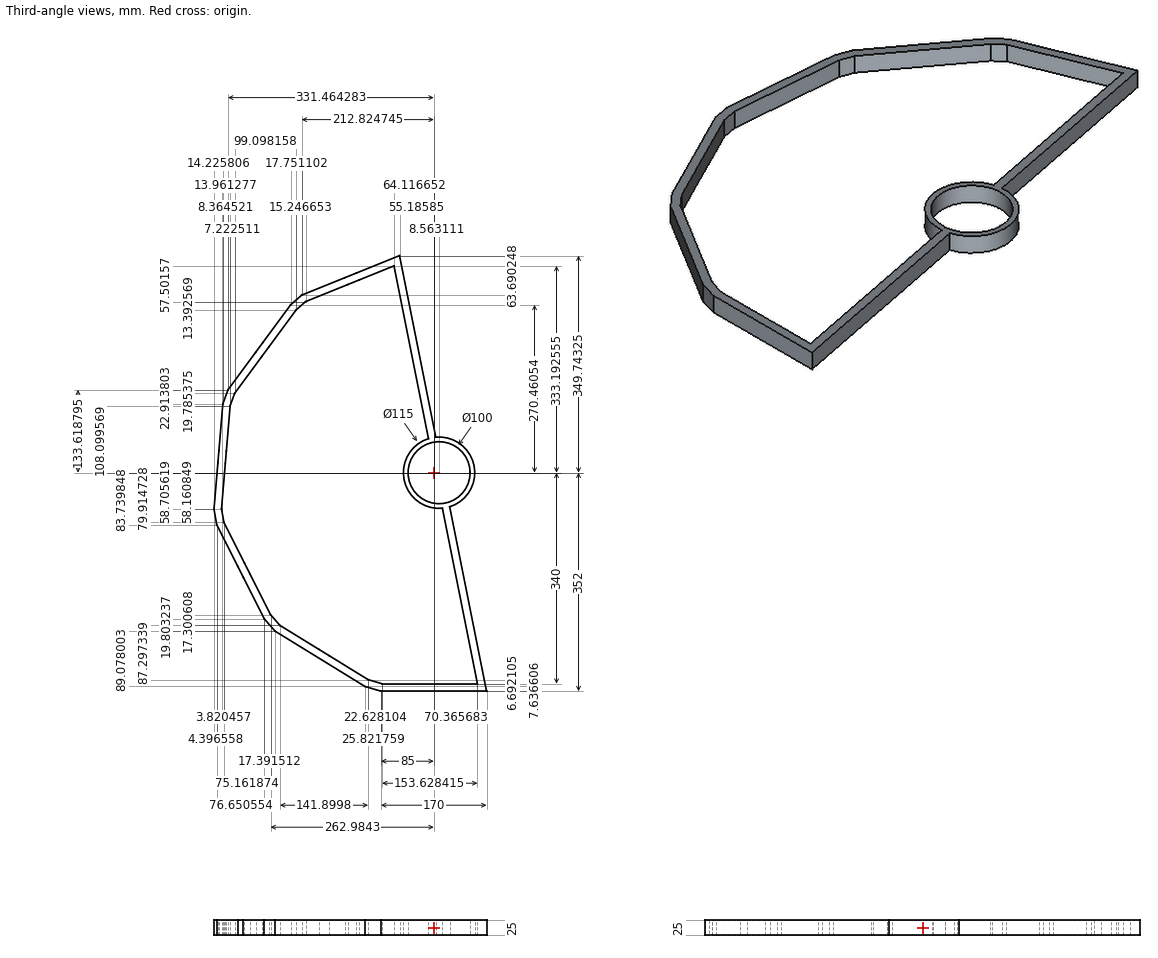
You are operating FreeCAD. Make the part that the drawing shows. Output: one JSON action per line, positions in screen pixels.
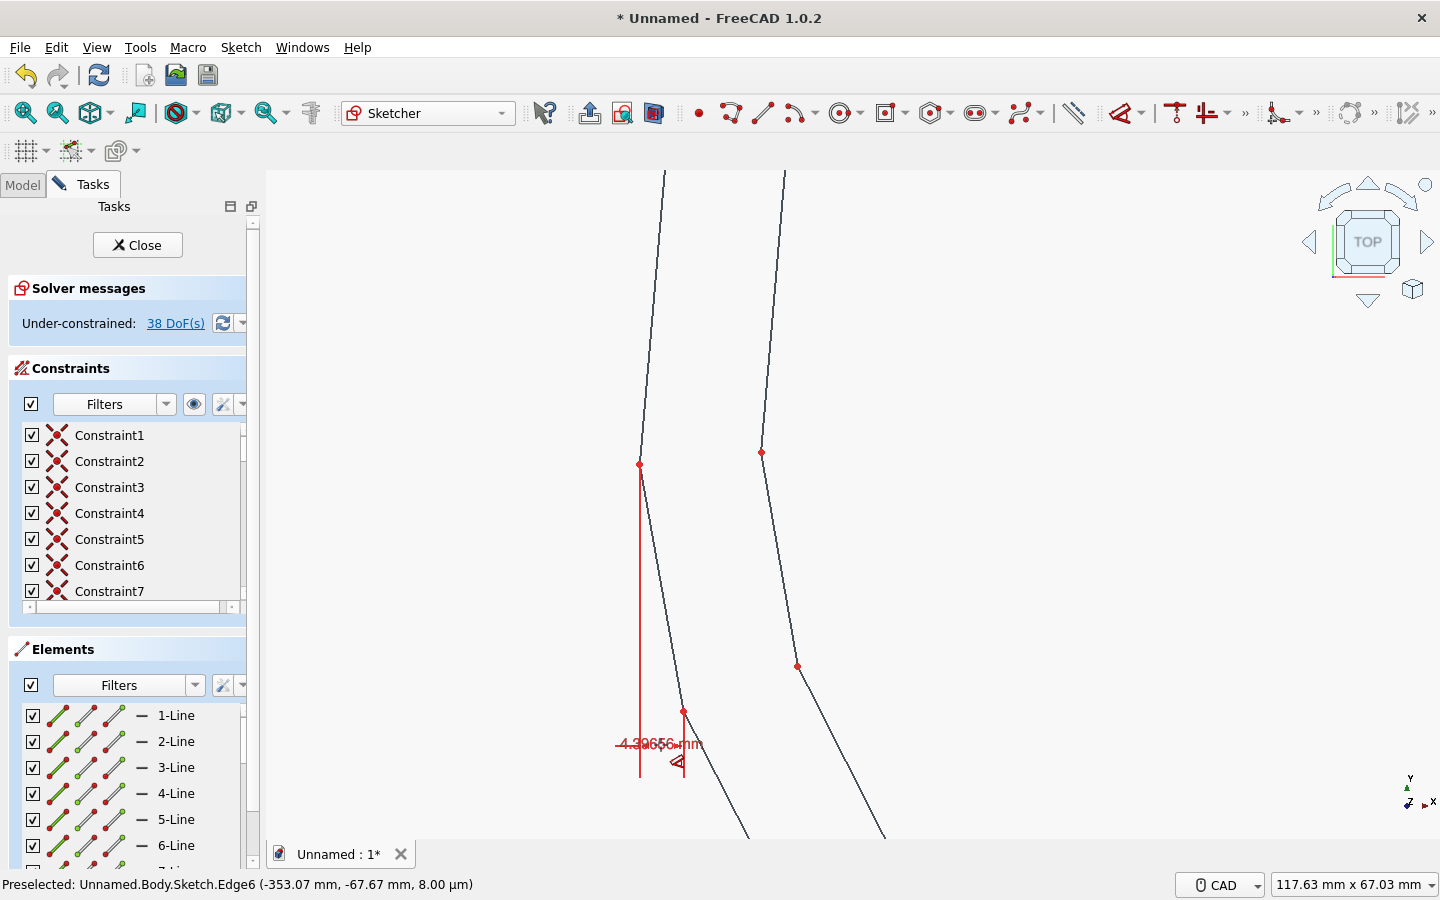
{"action": "scroll", "coordinate": [652, 545], "scroll_direction": "down", "scroll_amount": 14}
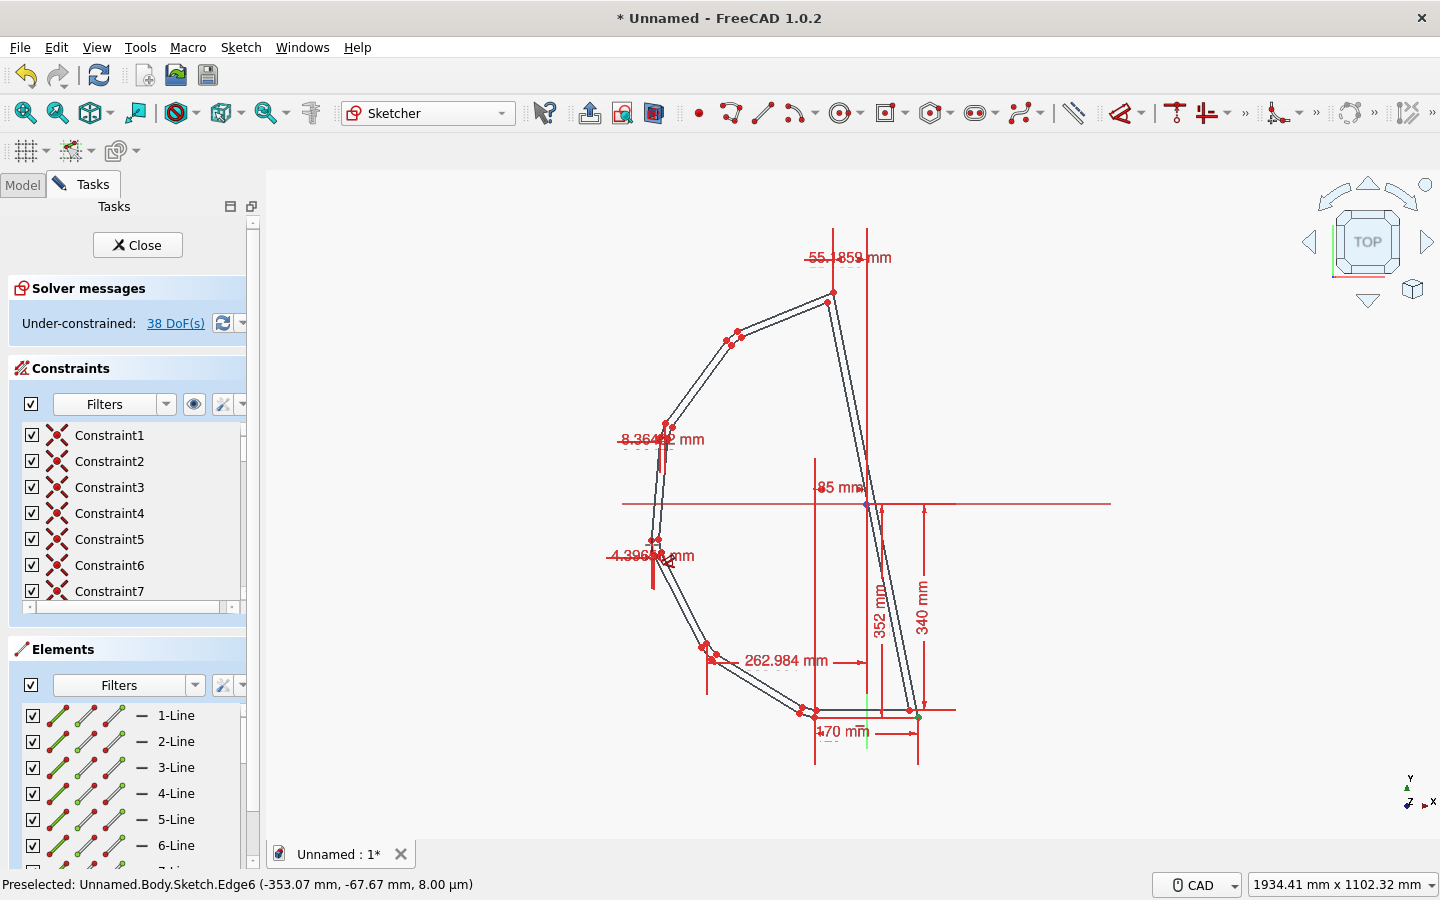
{"action": "scroll", "coordinate": [804, 715], "scroll_direction": "up", "scroll_amount": 11}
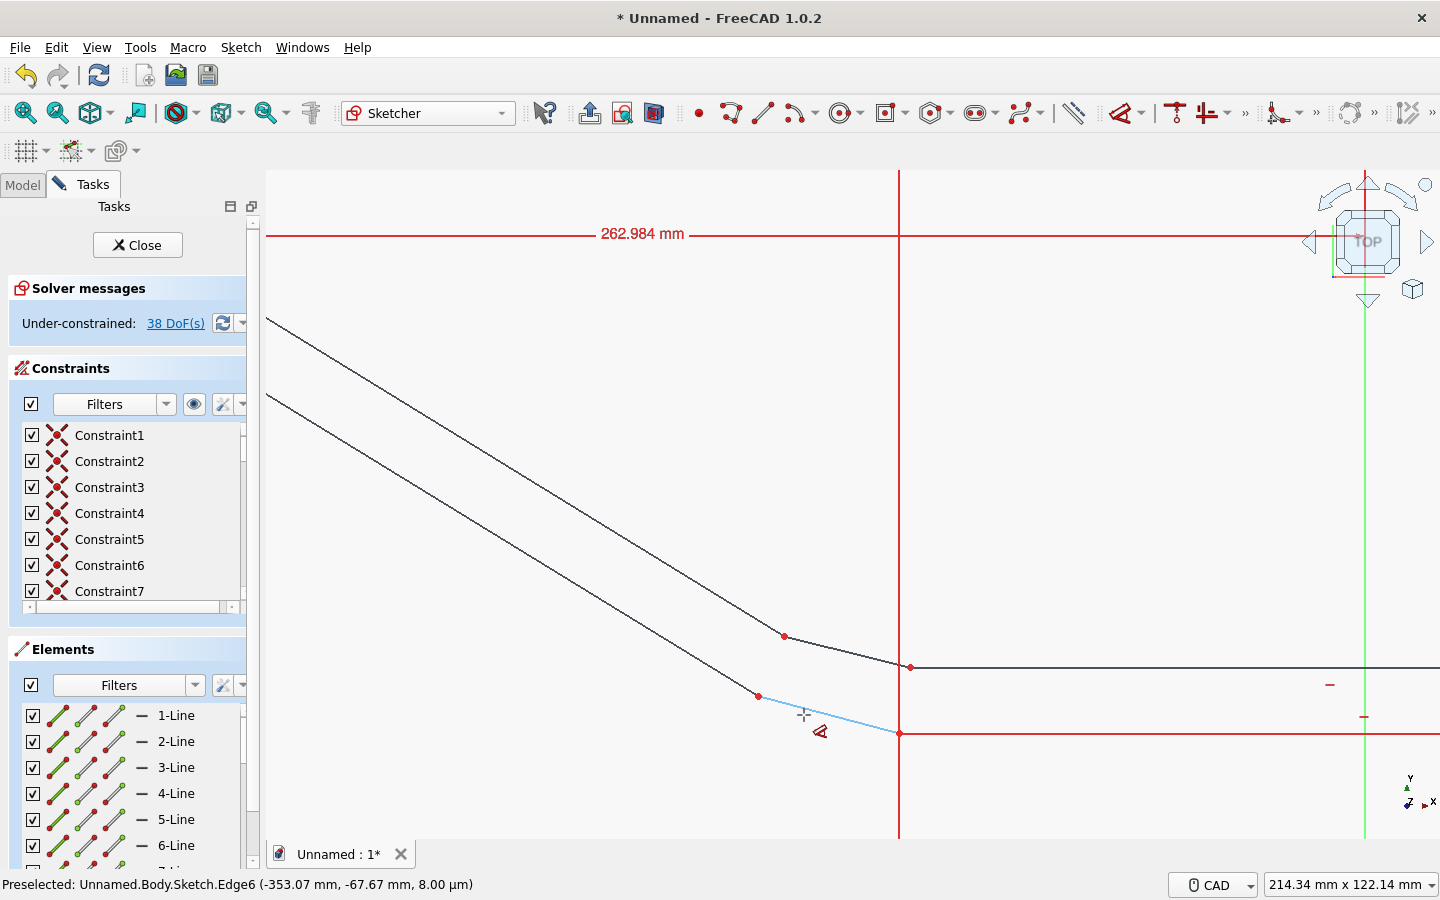
{"action": "left_click", "coordinate": [801, 707]}
{"action": "left_click", "coordinate": [933, 715]}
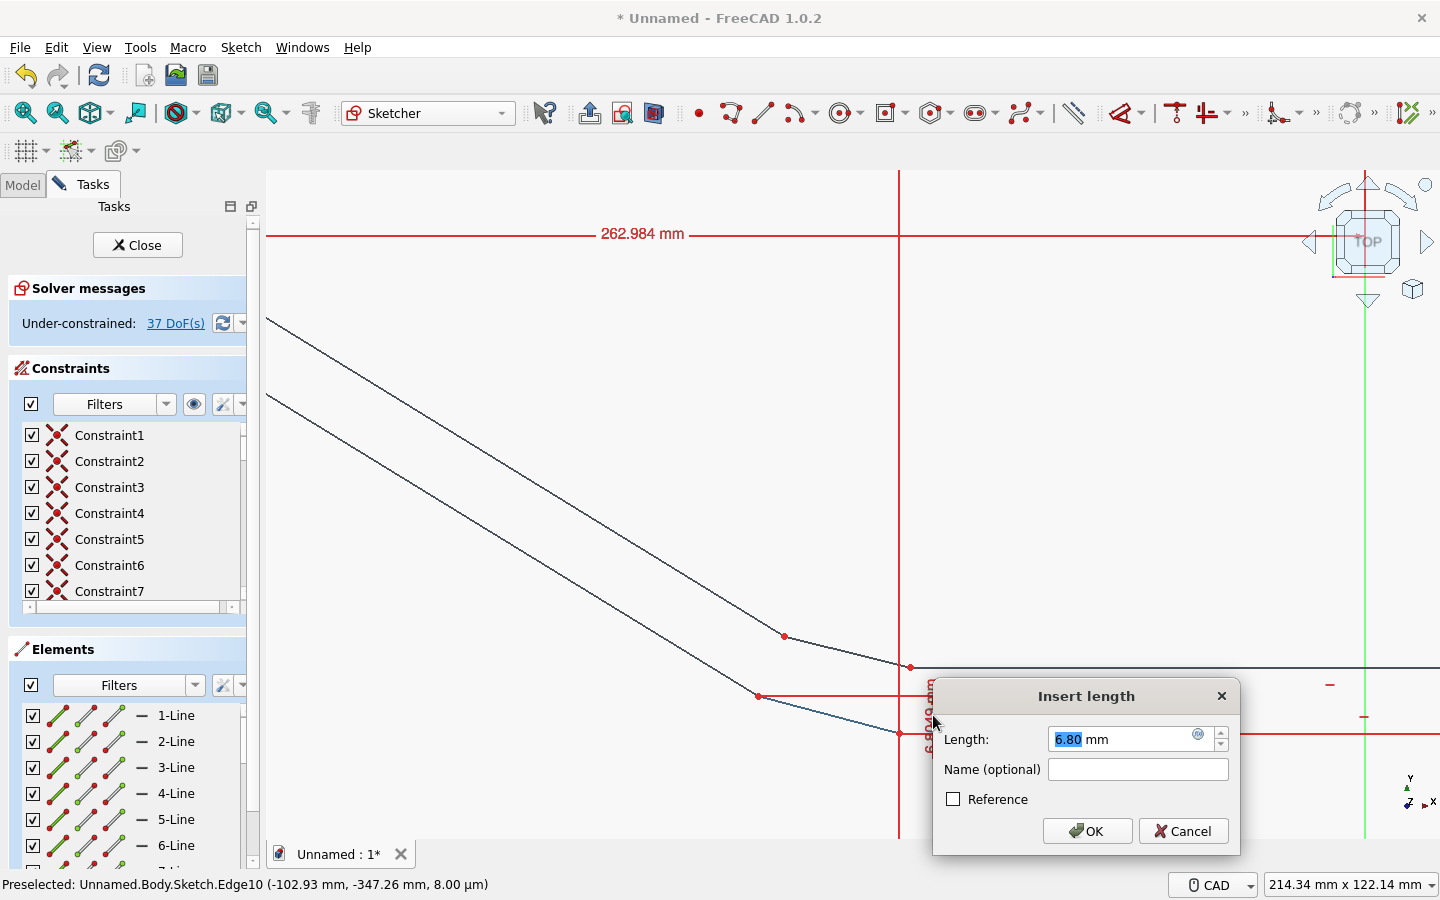
{"action": "type", "text": "7.636606"}
{"action": "key", "text": "Return"}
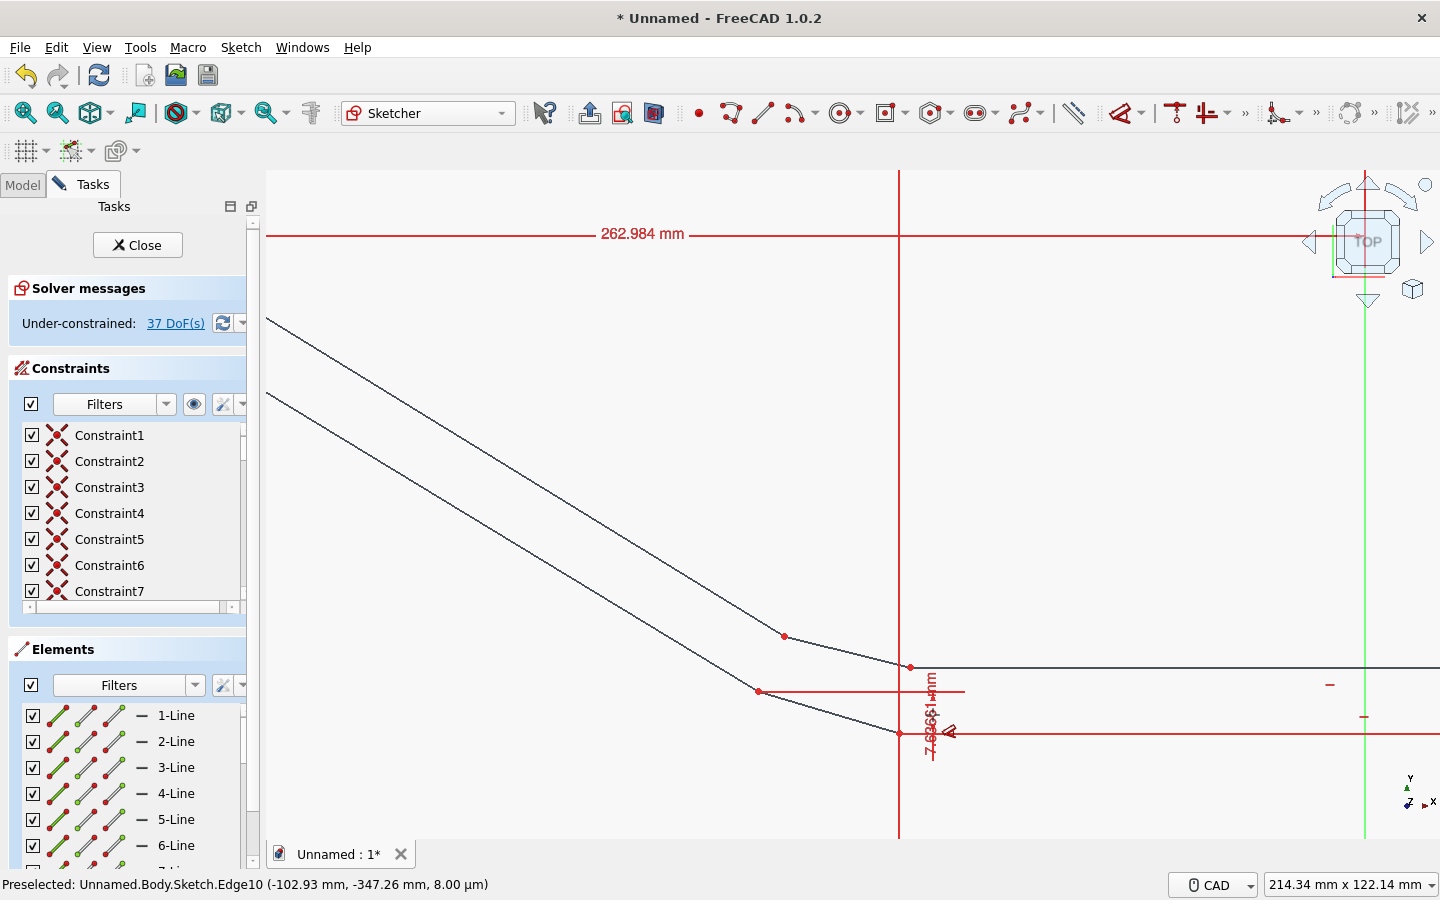
{"action": "left_click", "coordinate": [873, 658]}
{"action": "left_click", "coordinate": [944, 652]}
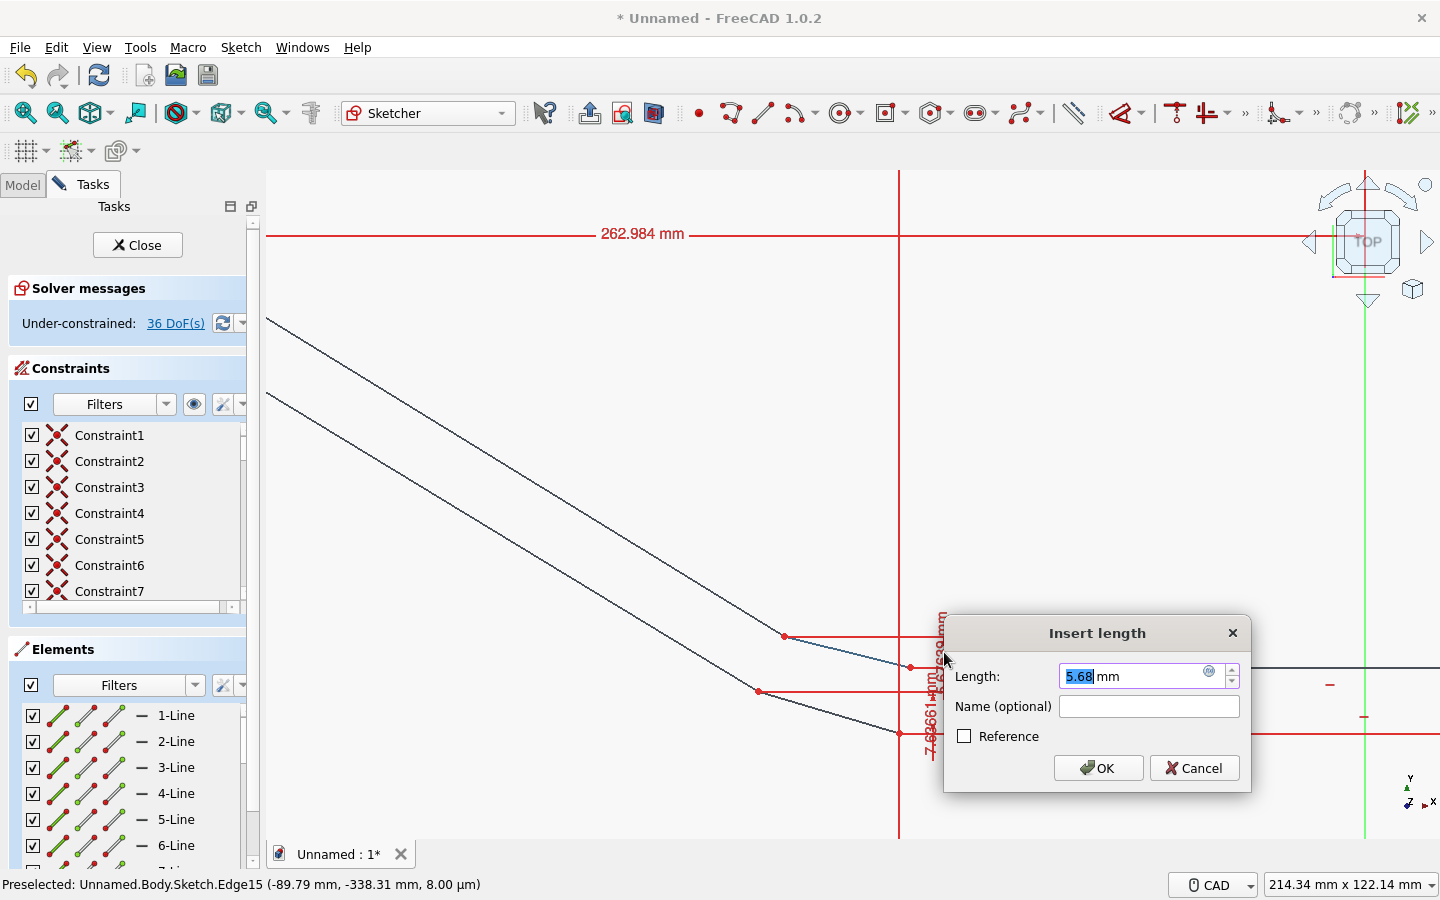
{"action": "type", "text": "6.692105"}
{"action": "key", "text": "Return"}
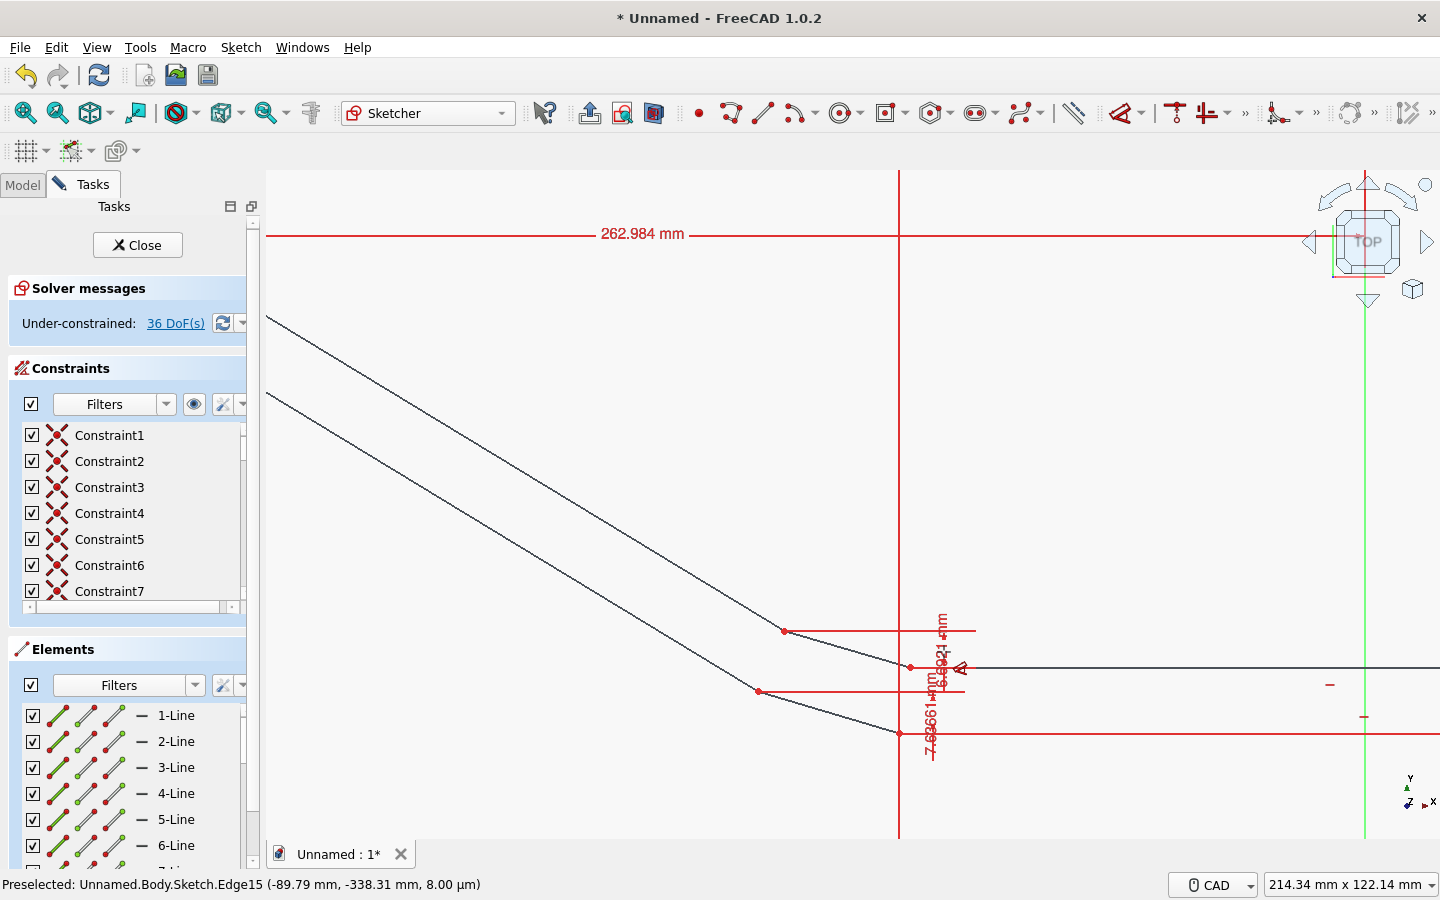
{"action": "scroll", "coordinate": [804, 715], "scroll_direction": "down", "scroll_amount": 11}